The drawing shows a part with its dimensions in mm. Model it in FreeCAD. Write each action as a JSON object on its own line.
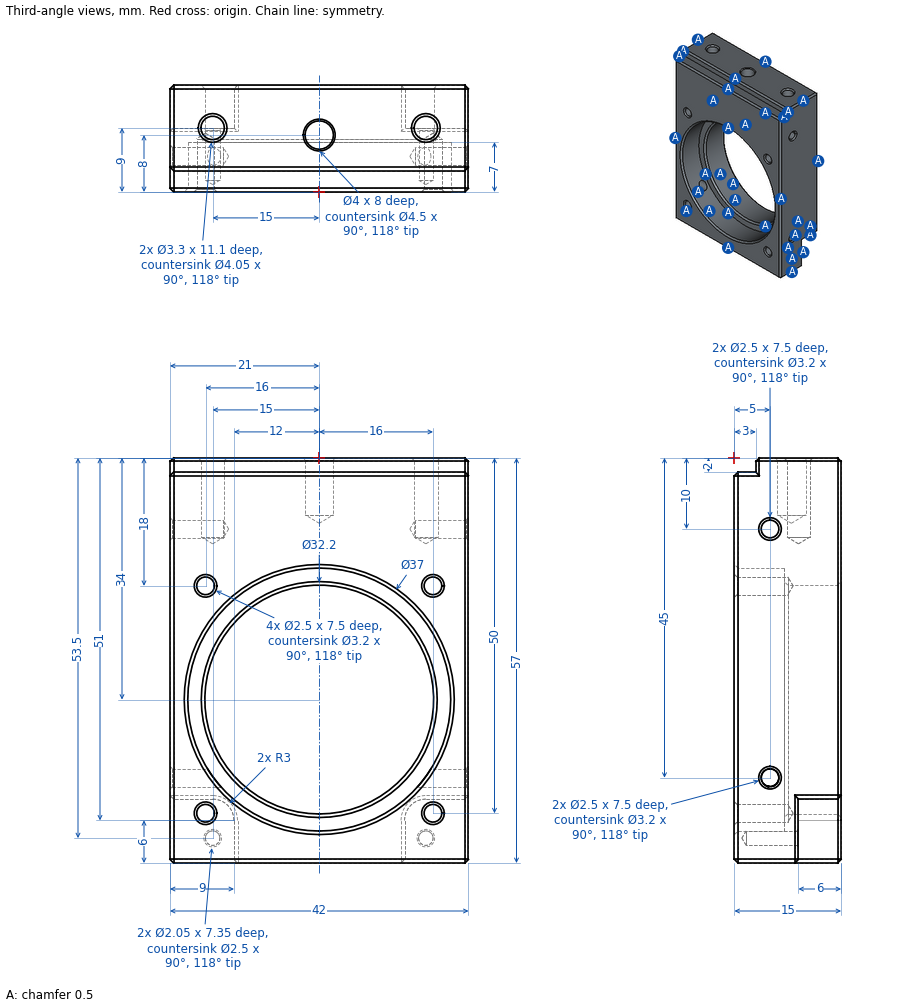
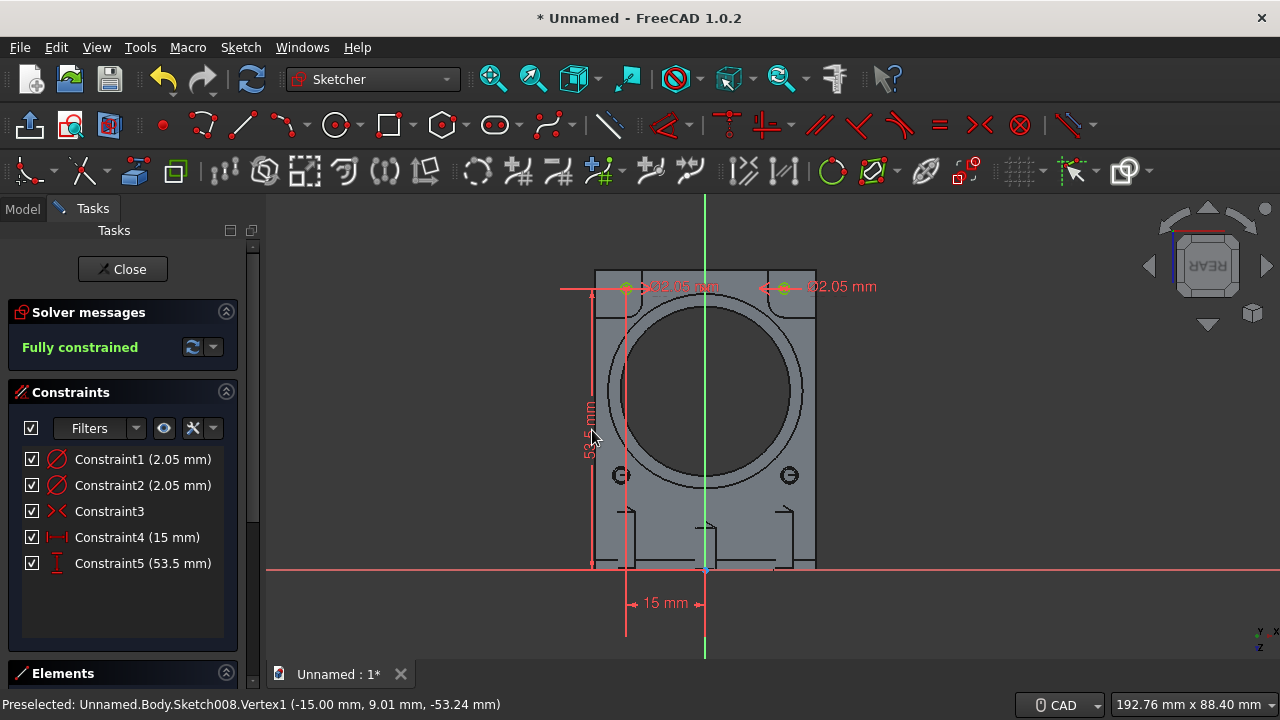
{"action": "left_click", "coordinate": [123, 269]}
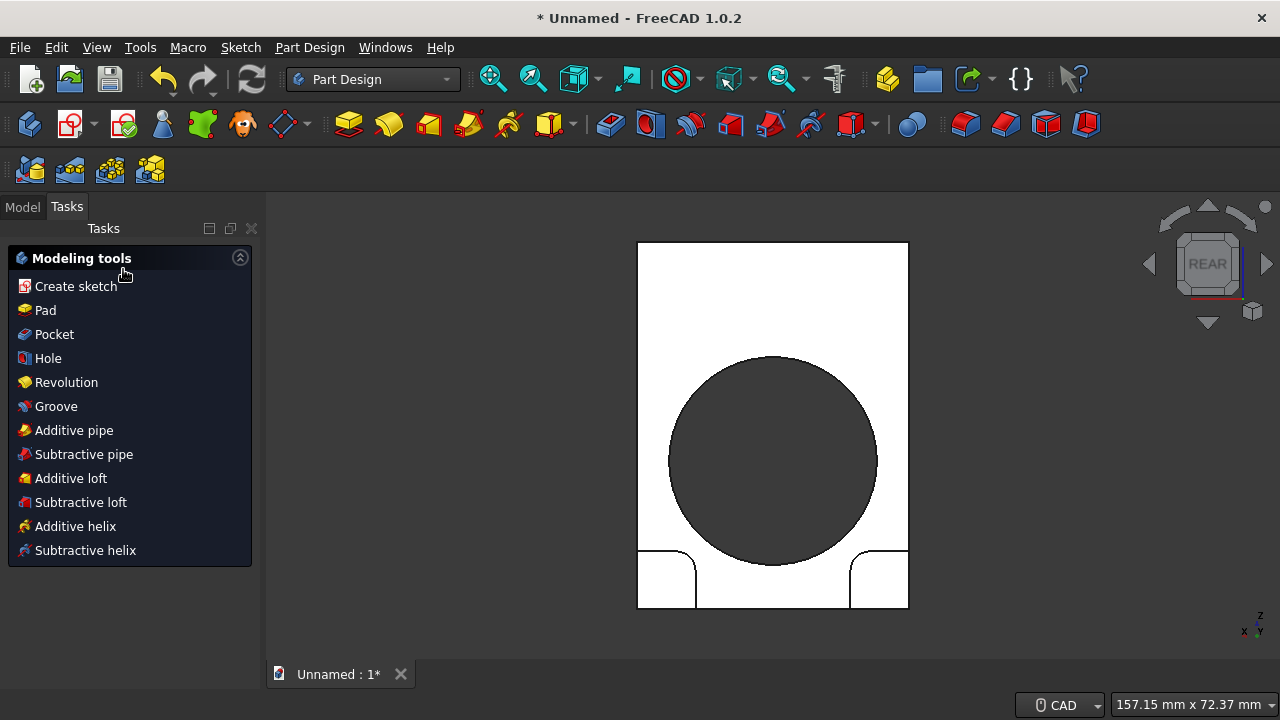
{"action": "left_click", "coordinate": [652, 124]}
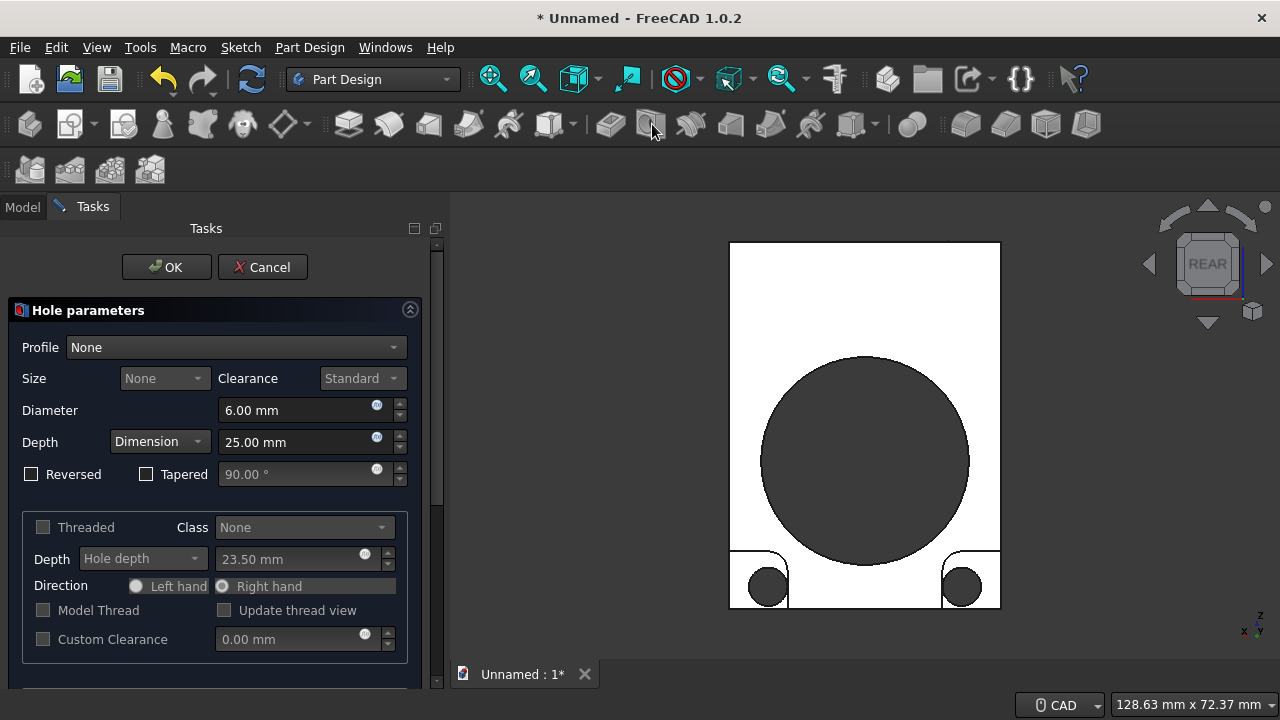
{"action": "triple_click", "coordinate": [305, 410]}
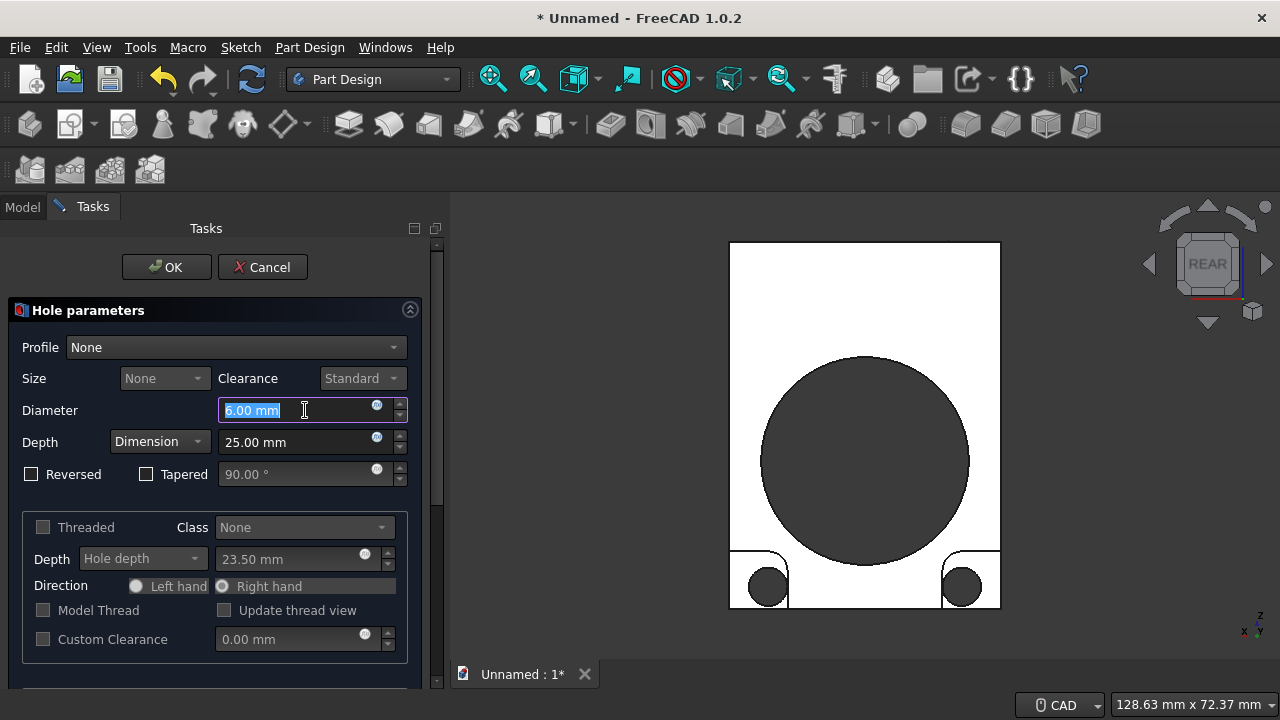
{"action": "type", "text": "2.05"}
{"action": "key", "text": "Tab"}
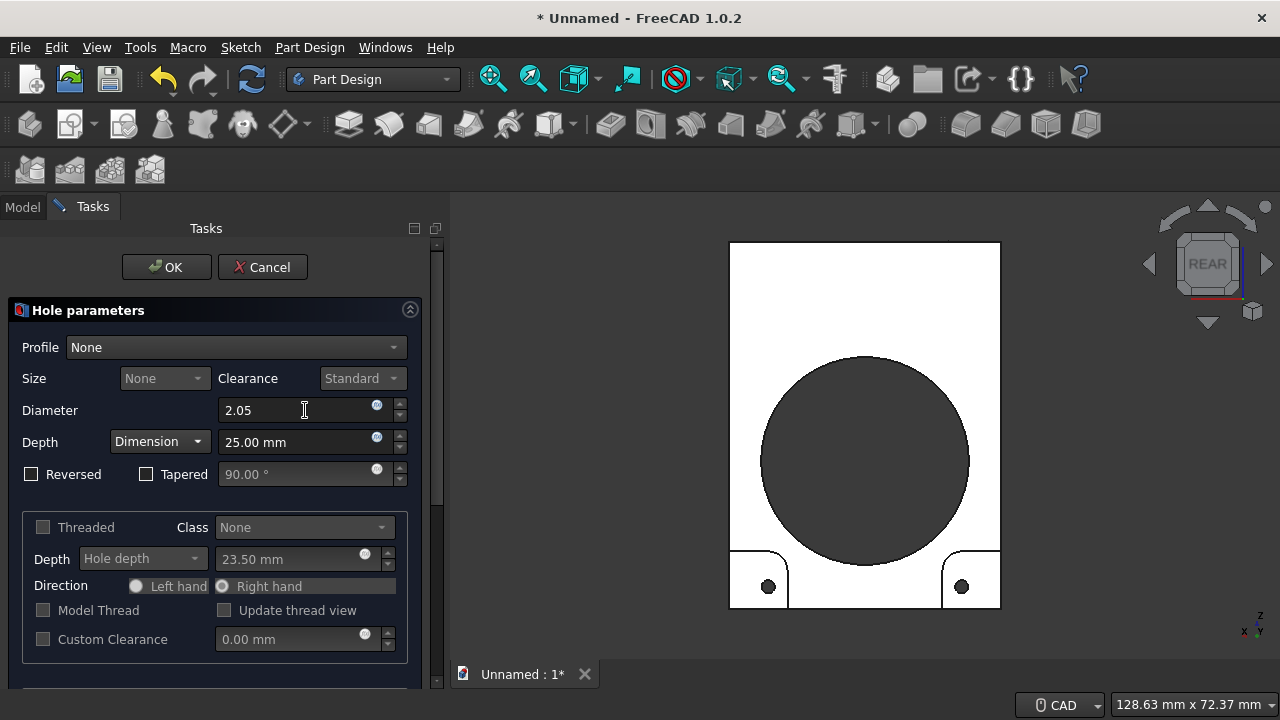
{"action": "triple_click", "coordinate": [305, 442]}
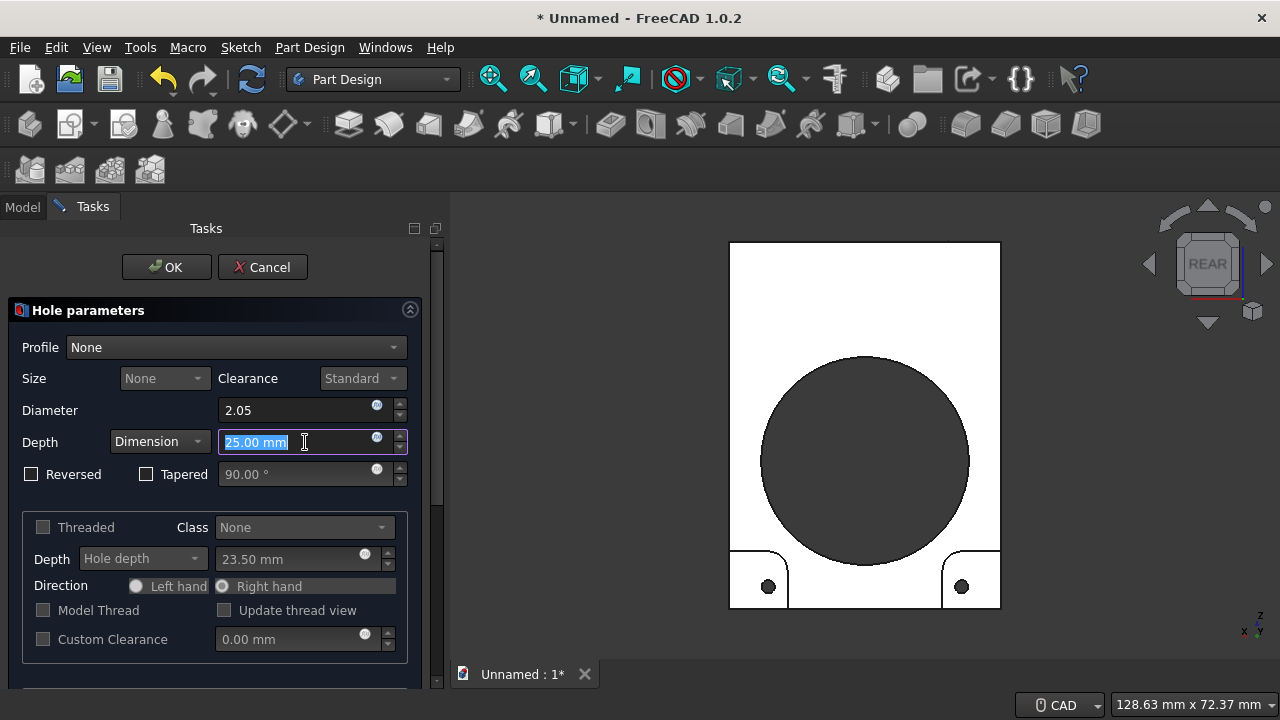
{"action": "type", "text": "7.35"}
{"action": "key", "text": "Tab"}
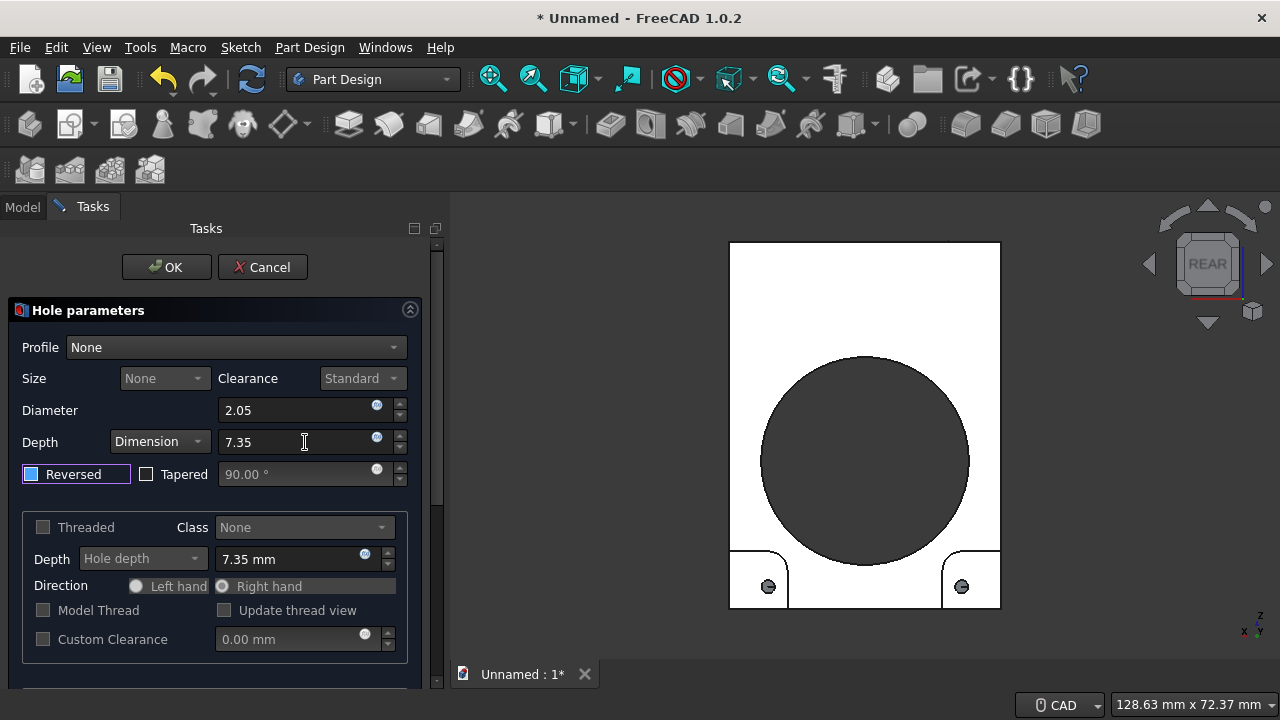
{"action": "scroll", "coordinate": [437, 463], "scroll_direction": "down", "scroll_amount": 2}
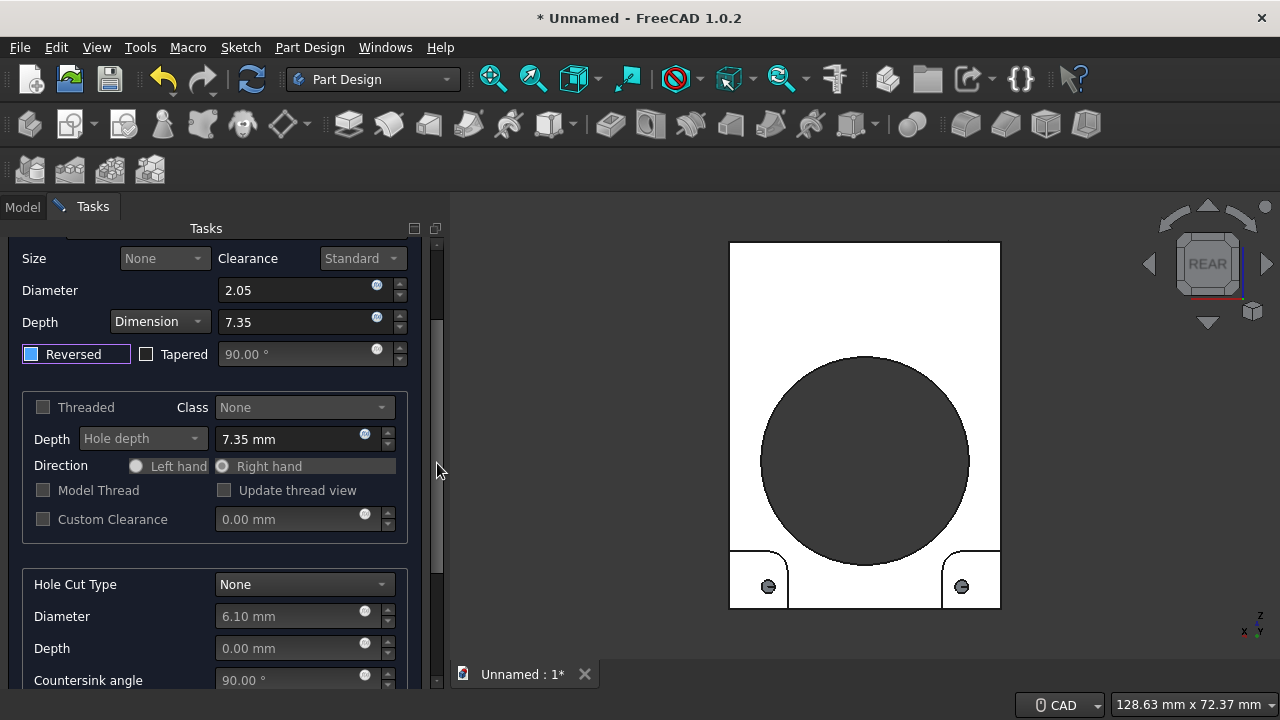
{"action": "left_click", "coordinate": [306, 584]}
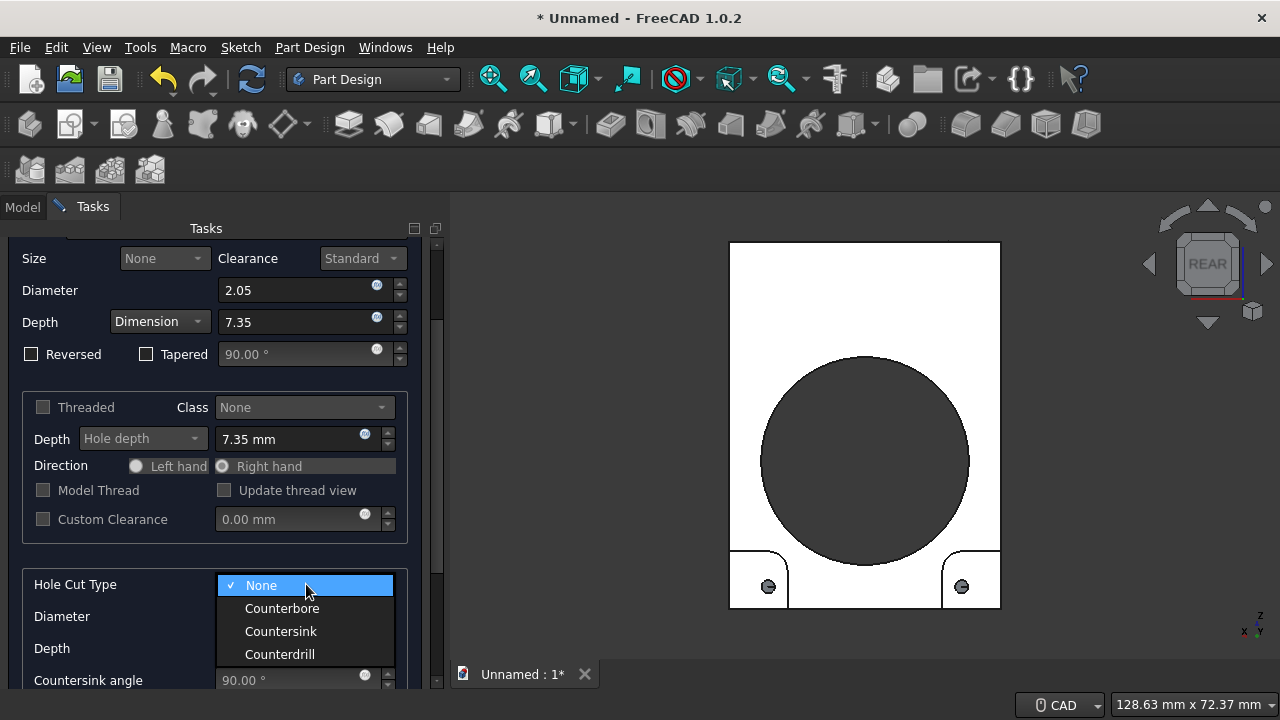
{"action": "left_click", "coordinate": [304, 632]}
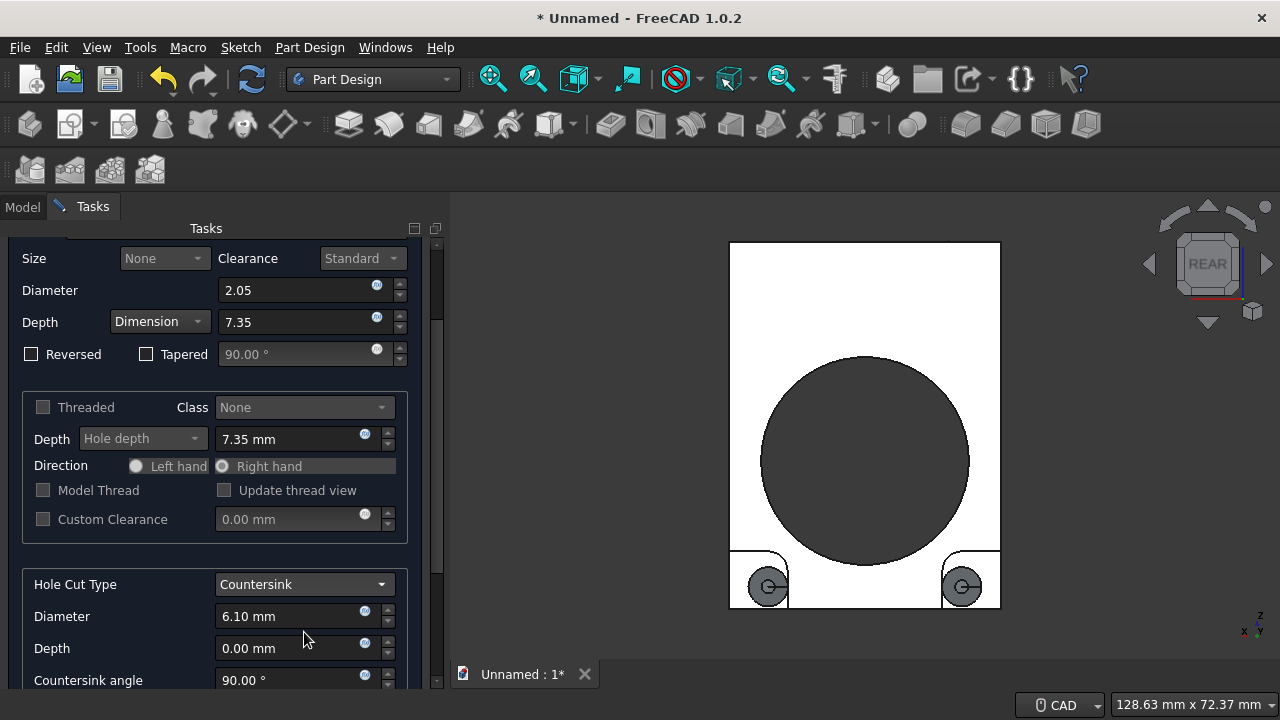
{"action": "triple_click", "coordinate": [298, 616]}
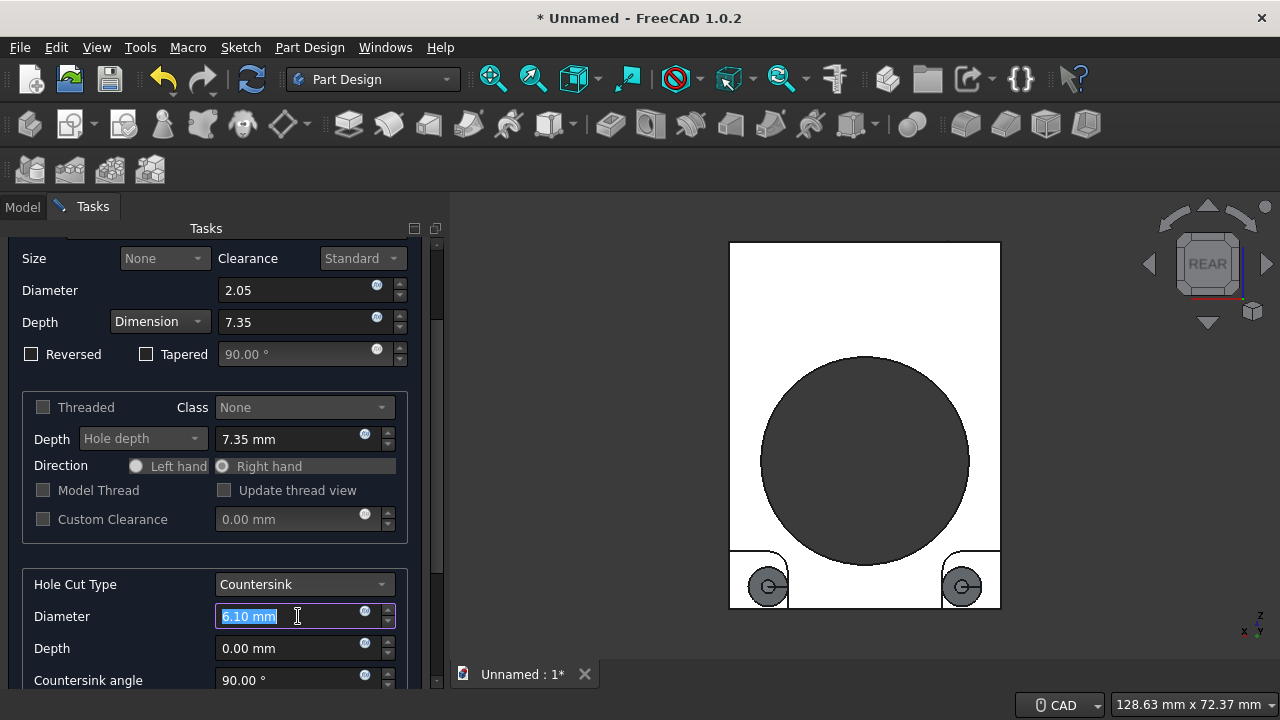
{"action": "type", "text": "2.5"}
{"action": "key", "text": "Tab"}